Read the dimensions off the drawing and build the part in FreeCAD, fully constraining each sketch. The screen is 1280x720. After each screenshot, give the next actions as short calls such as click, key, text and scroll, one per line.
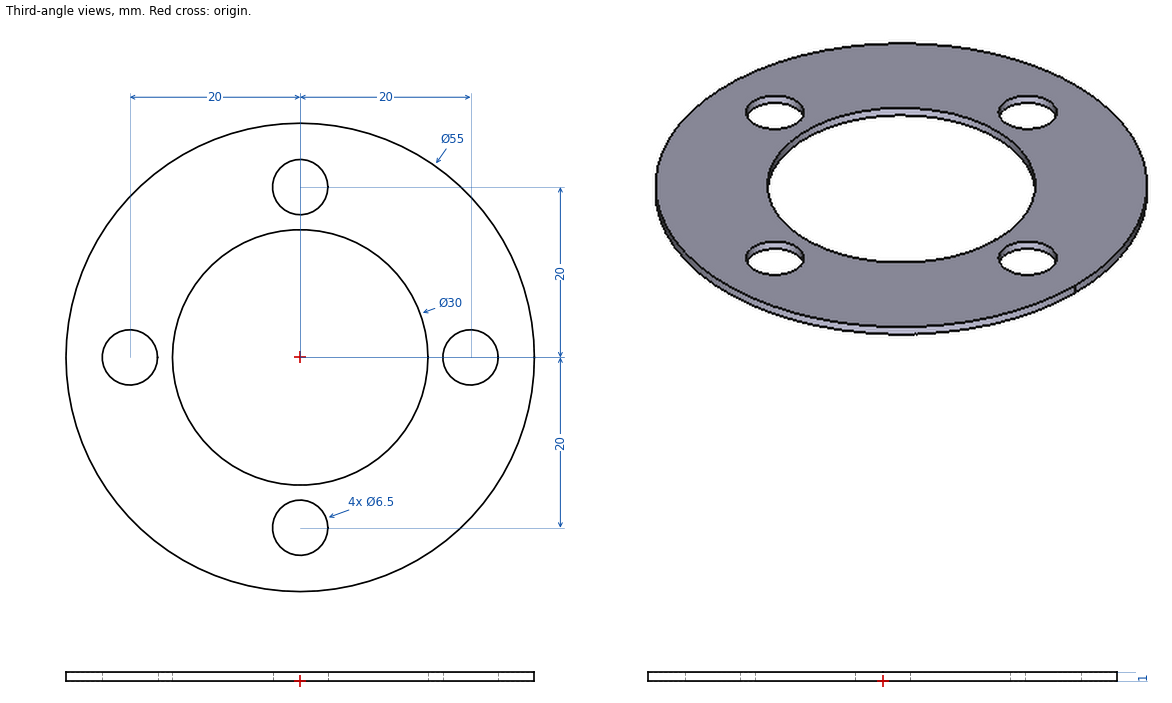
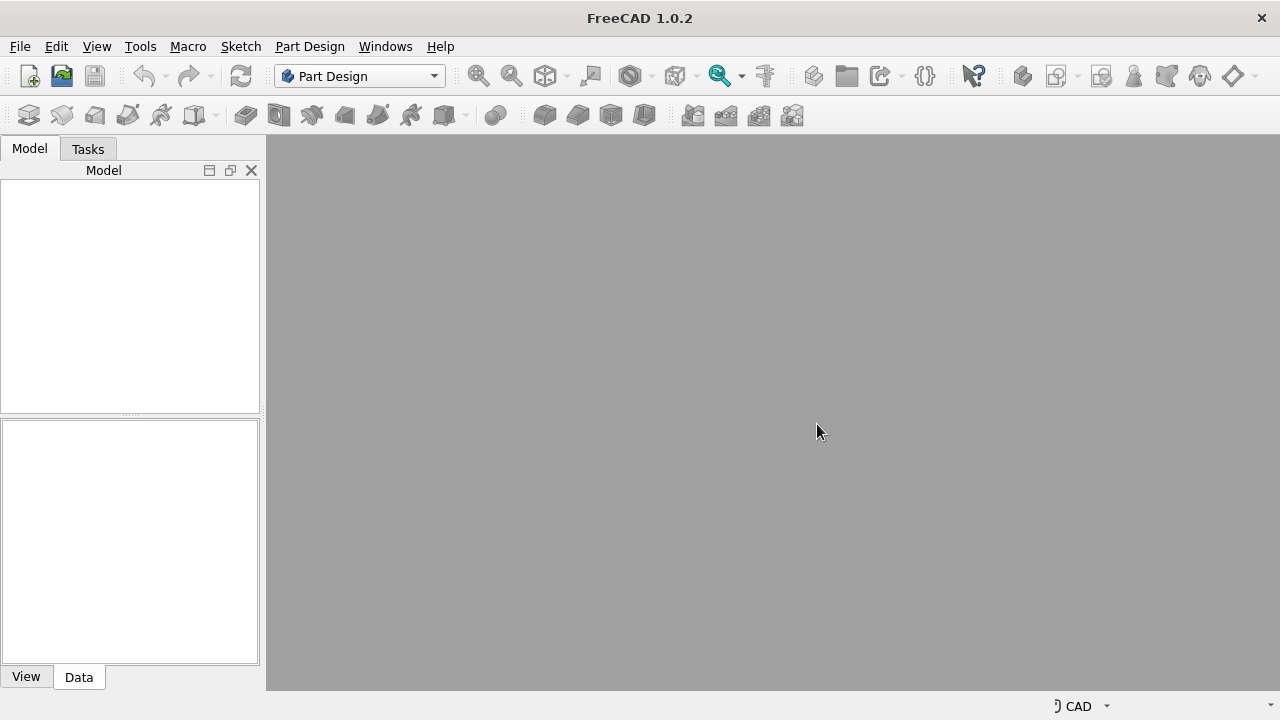
click(29, 76)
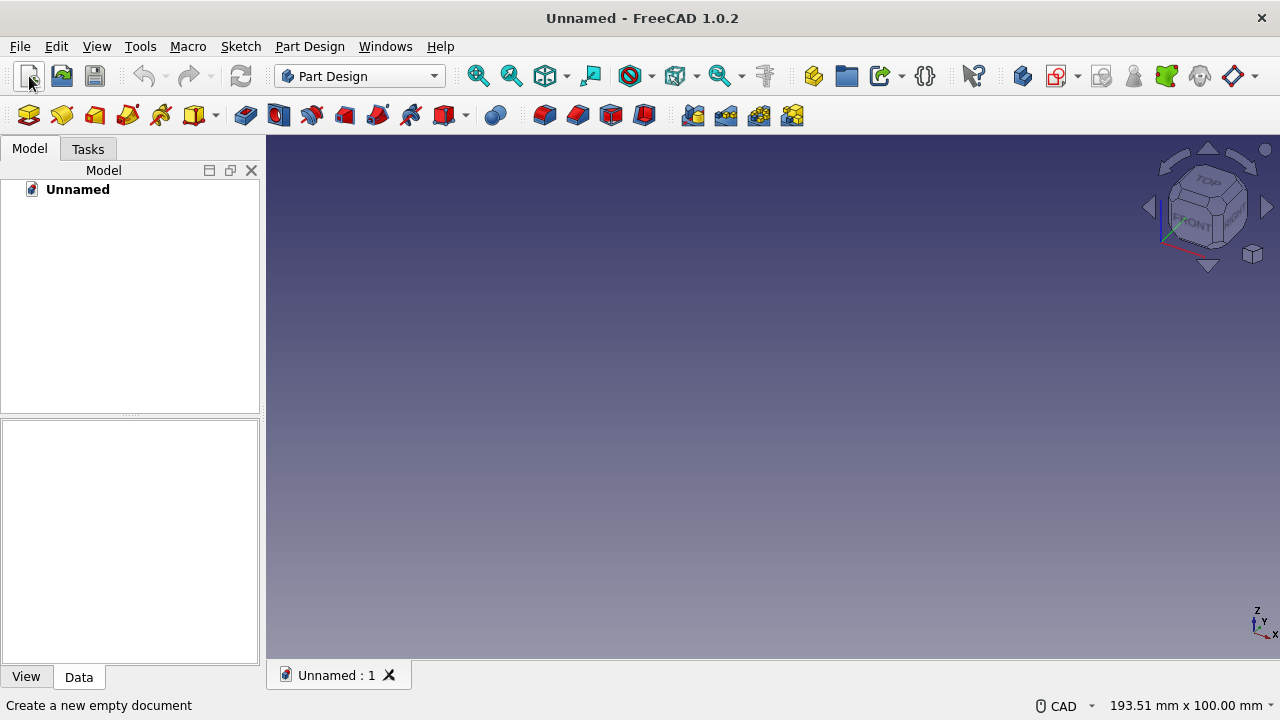
click(1056, 76)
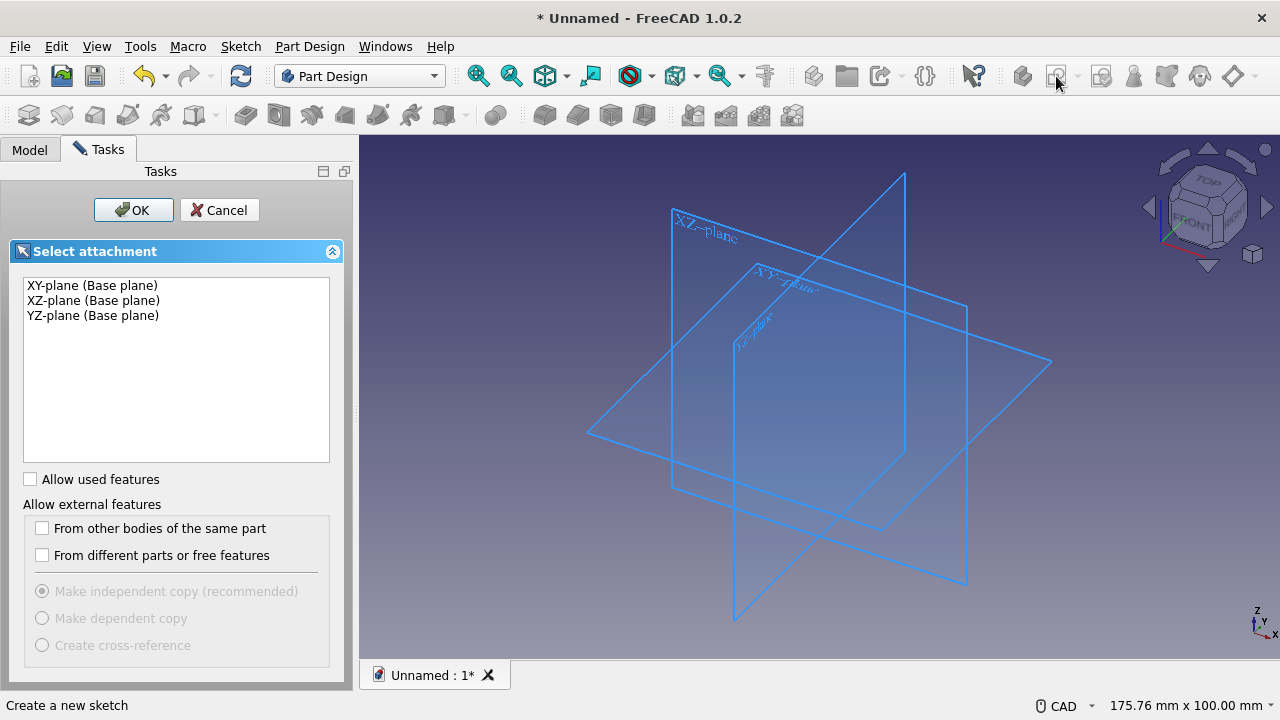
click(84, 286)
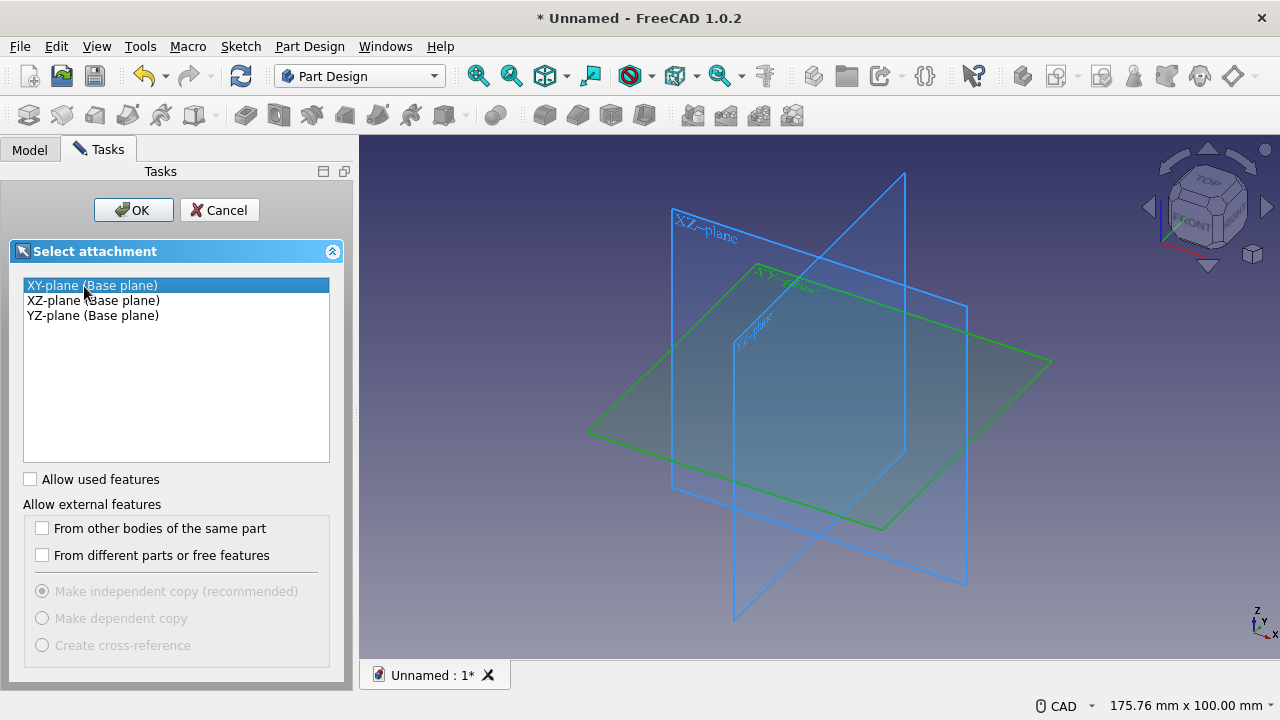
click(134, 210)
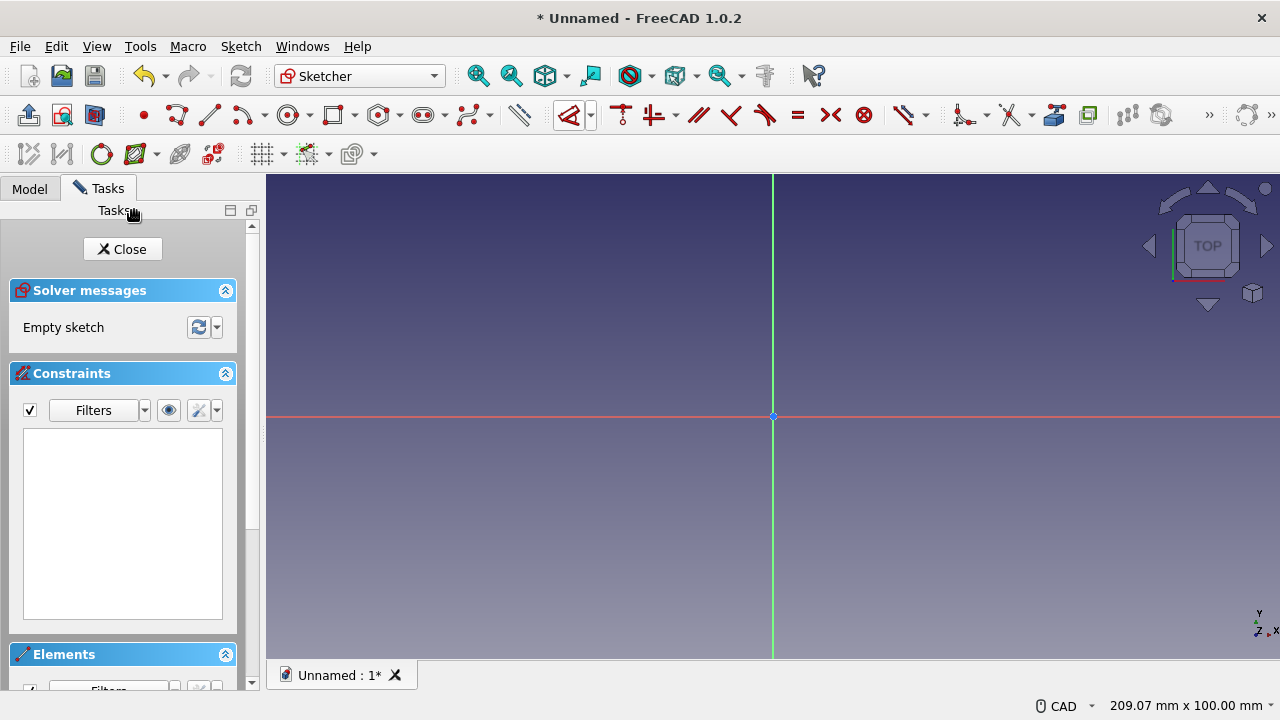
key(g)
key(c)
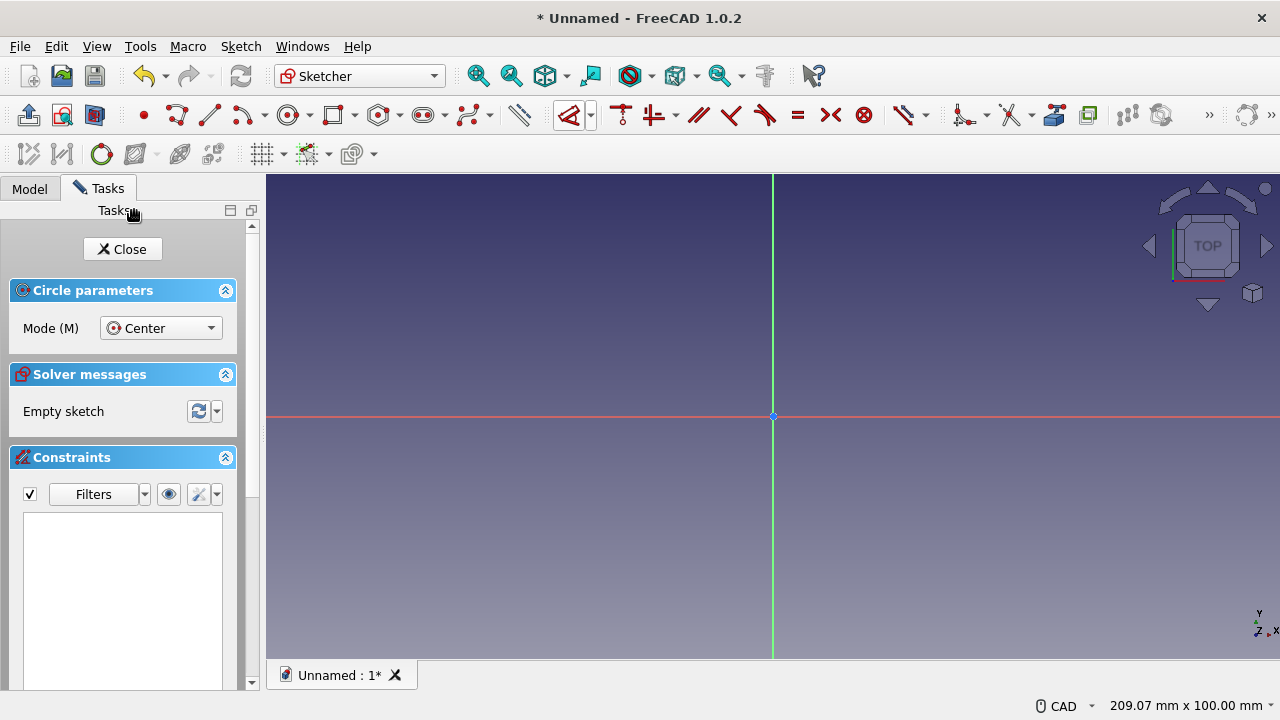
click(773, 416)
click(867, 322)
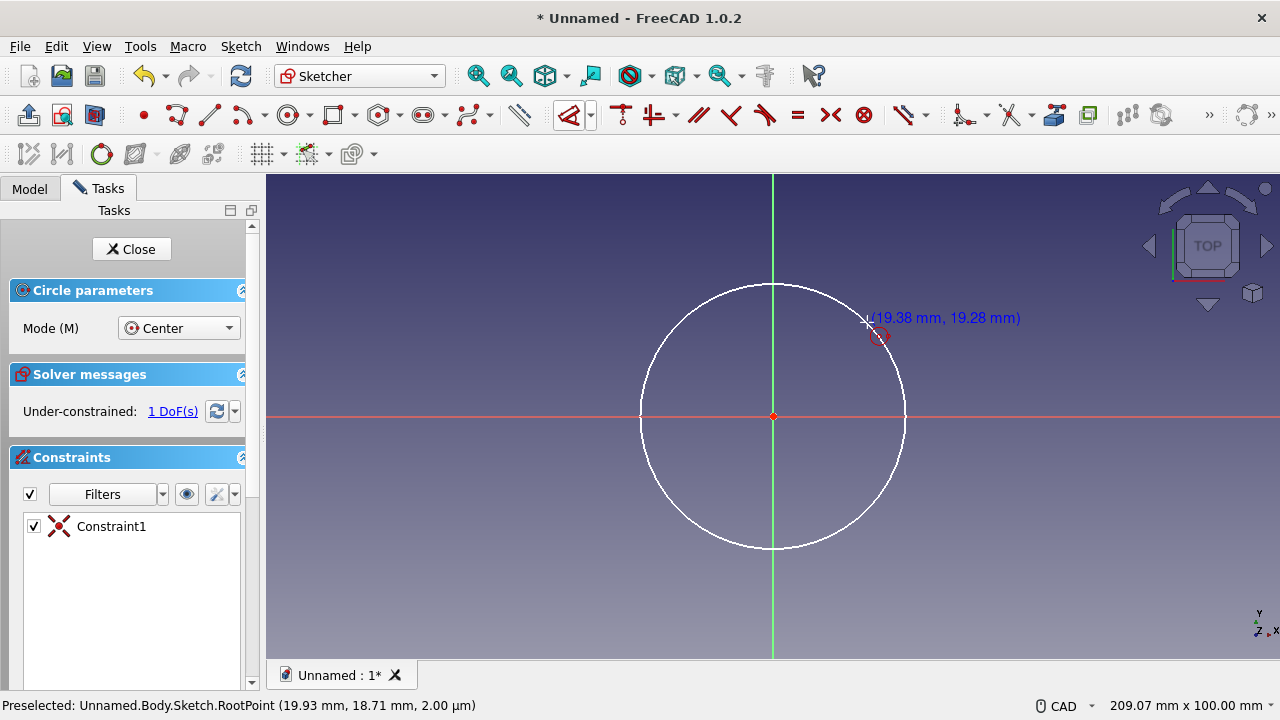
scroll(773, 514, up, 2)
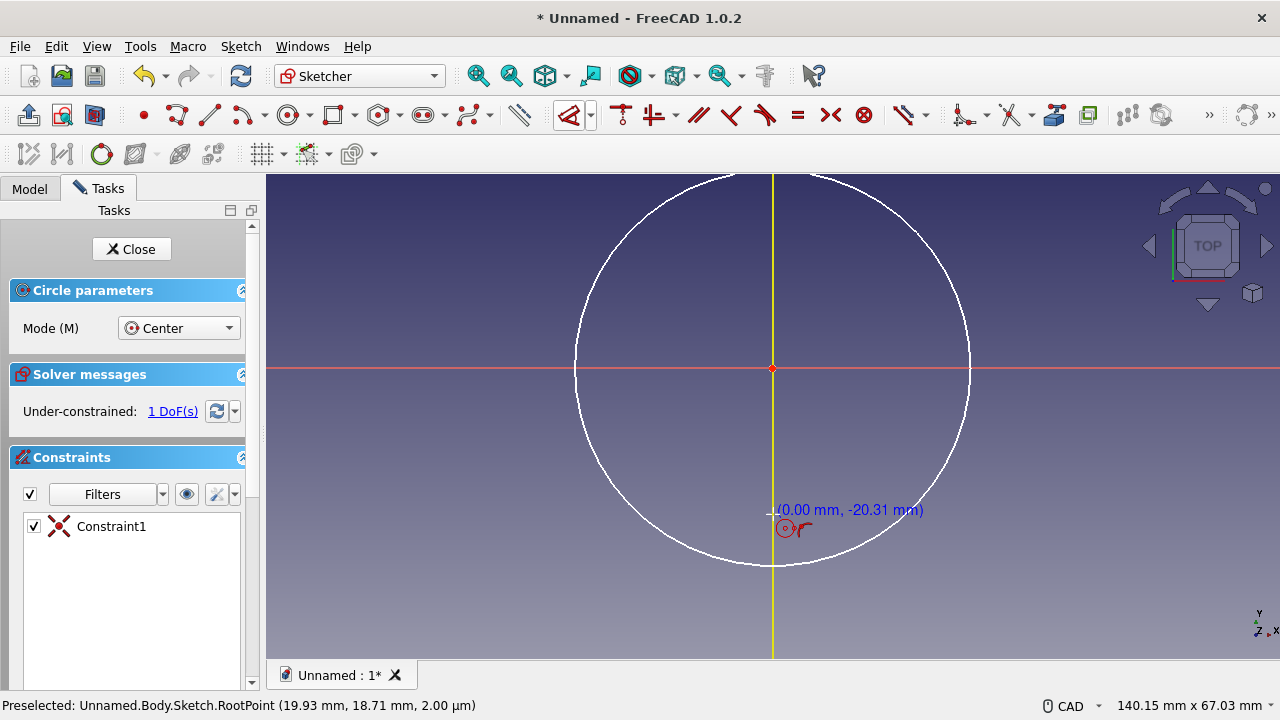
click(773, 513)
click(789, 496)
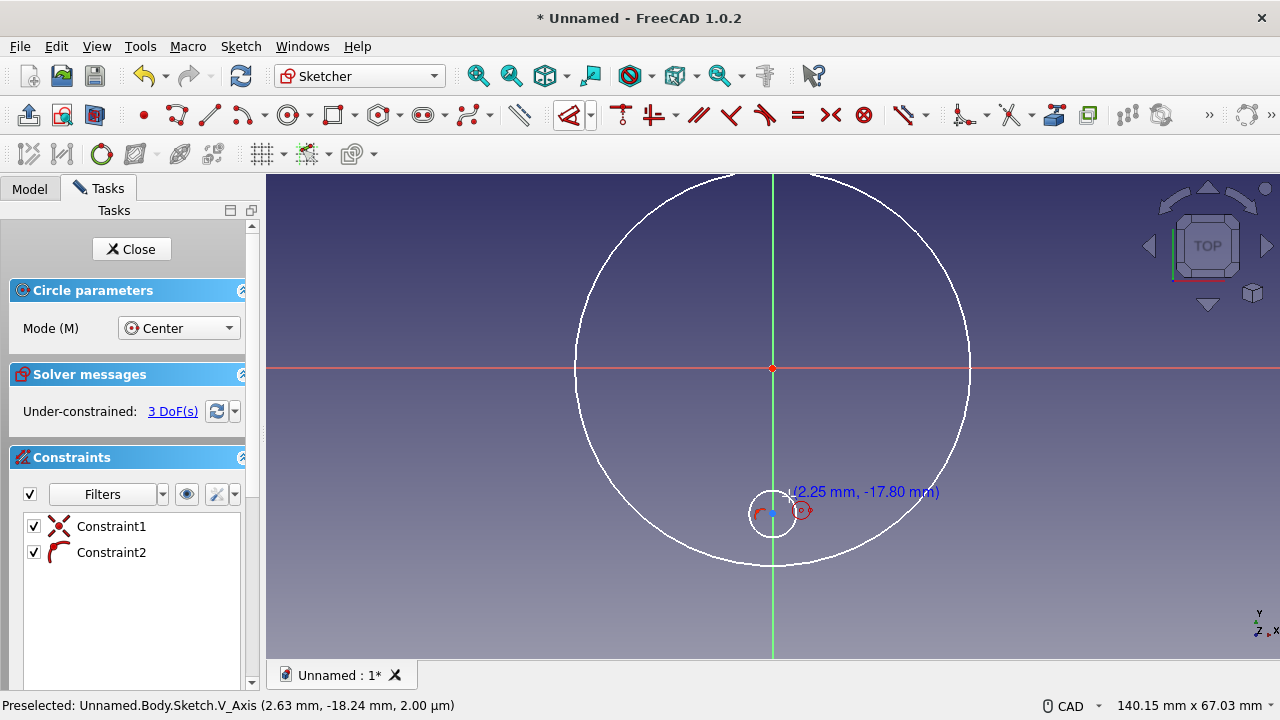
click(628, 368)
click(645, 352)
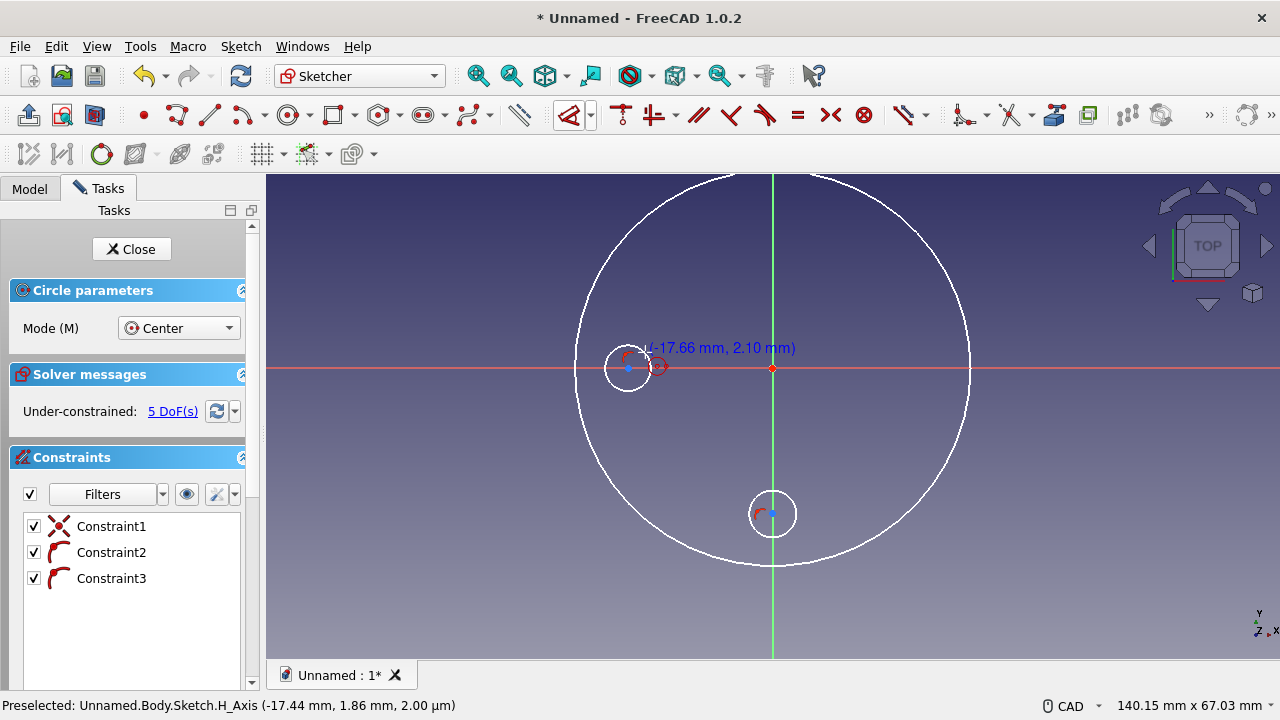
click(773, 368)
click(849, 291)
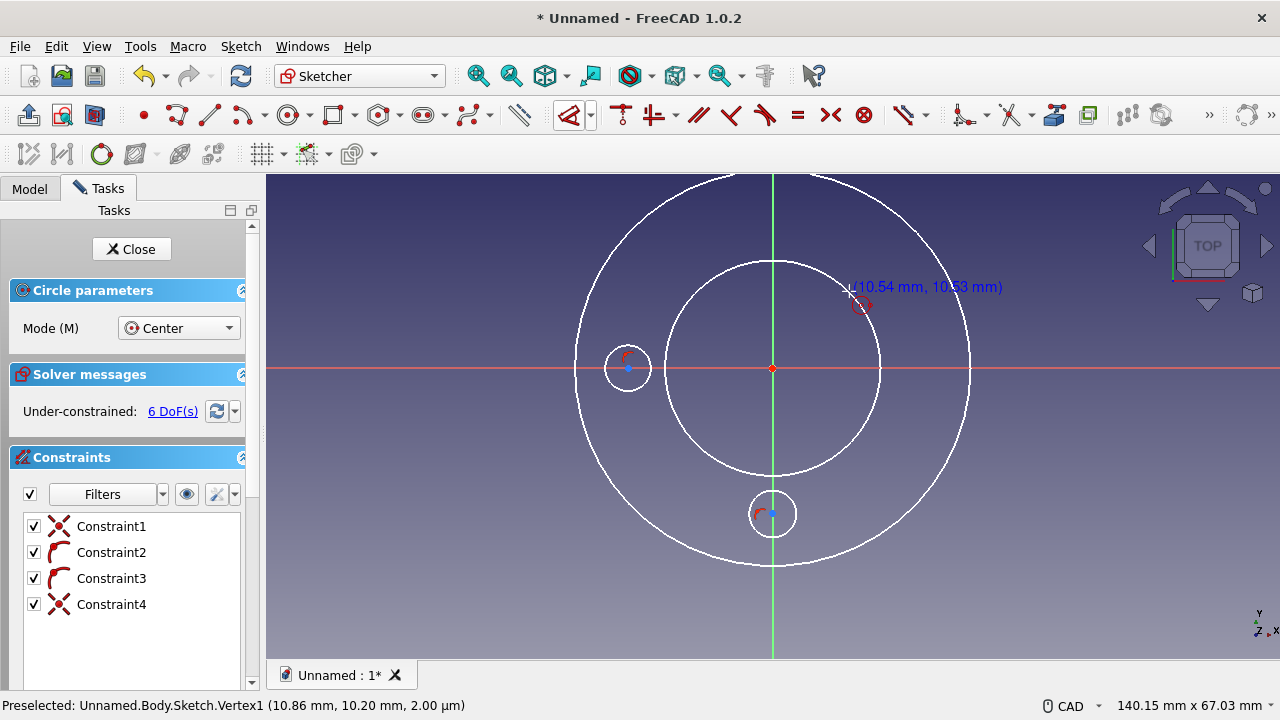
click(917, 368)
click(934, 352)